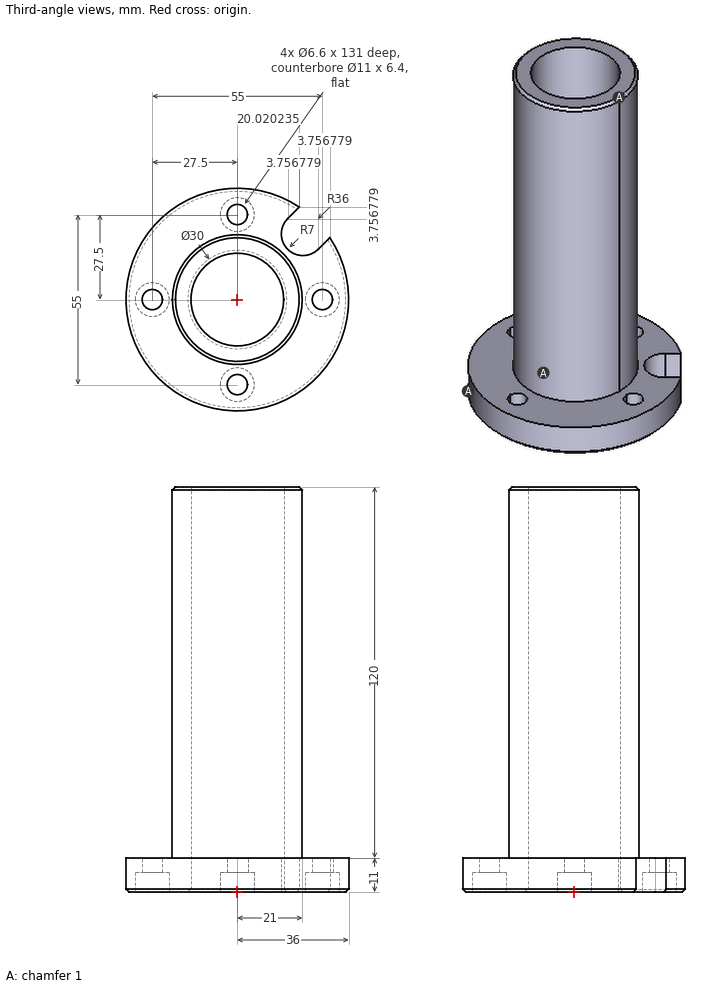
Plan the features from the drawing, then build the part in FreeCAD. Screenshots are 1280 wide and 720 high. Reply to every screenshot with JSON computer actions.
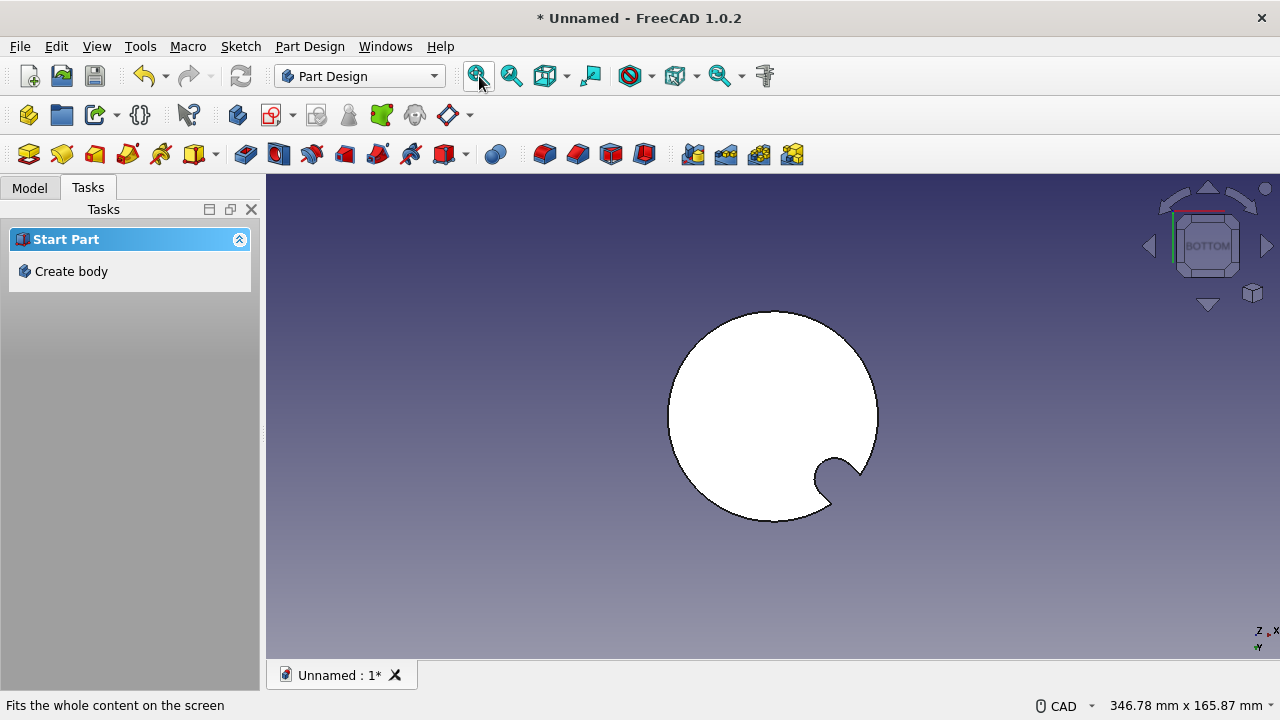
{"action": "left_click", "coordinate": [479, 76]}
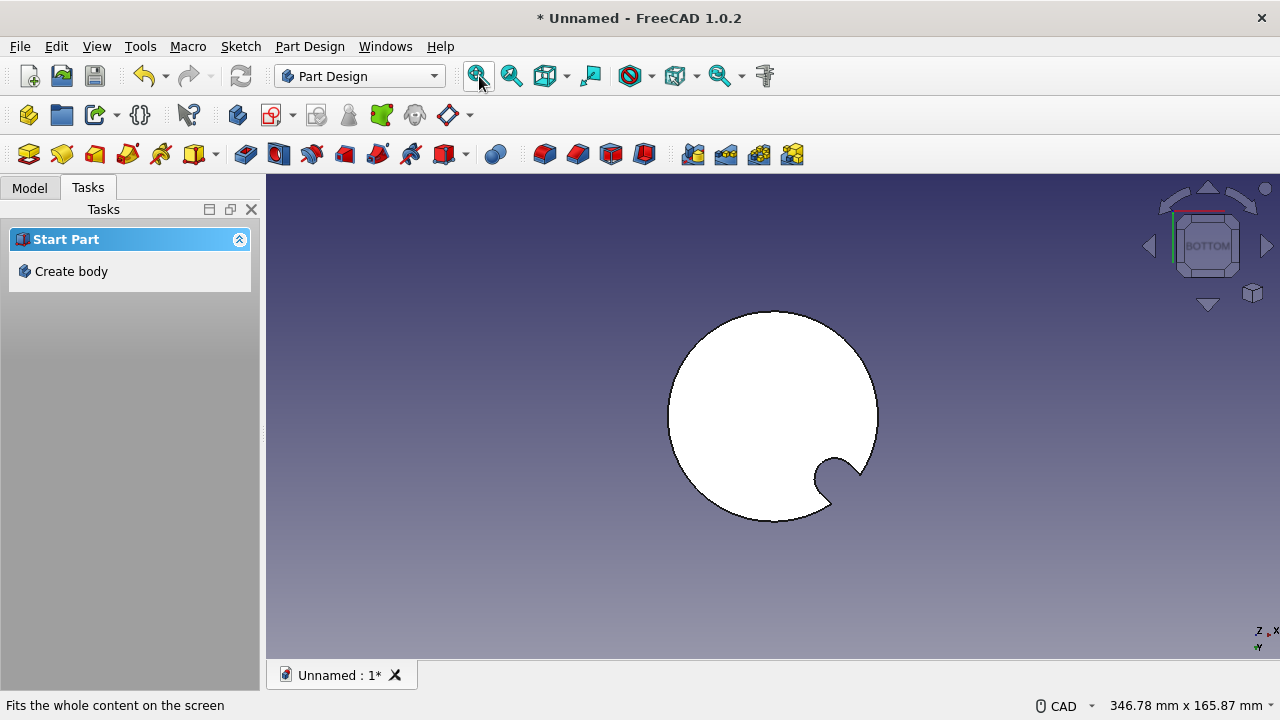
{"action": "left_click", "coordinate": [773, 385]}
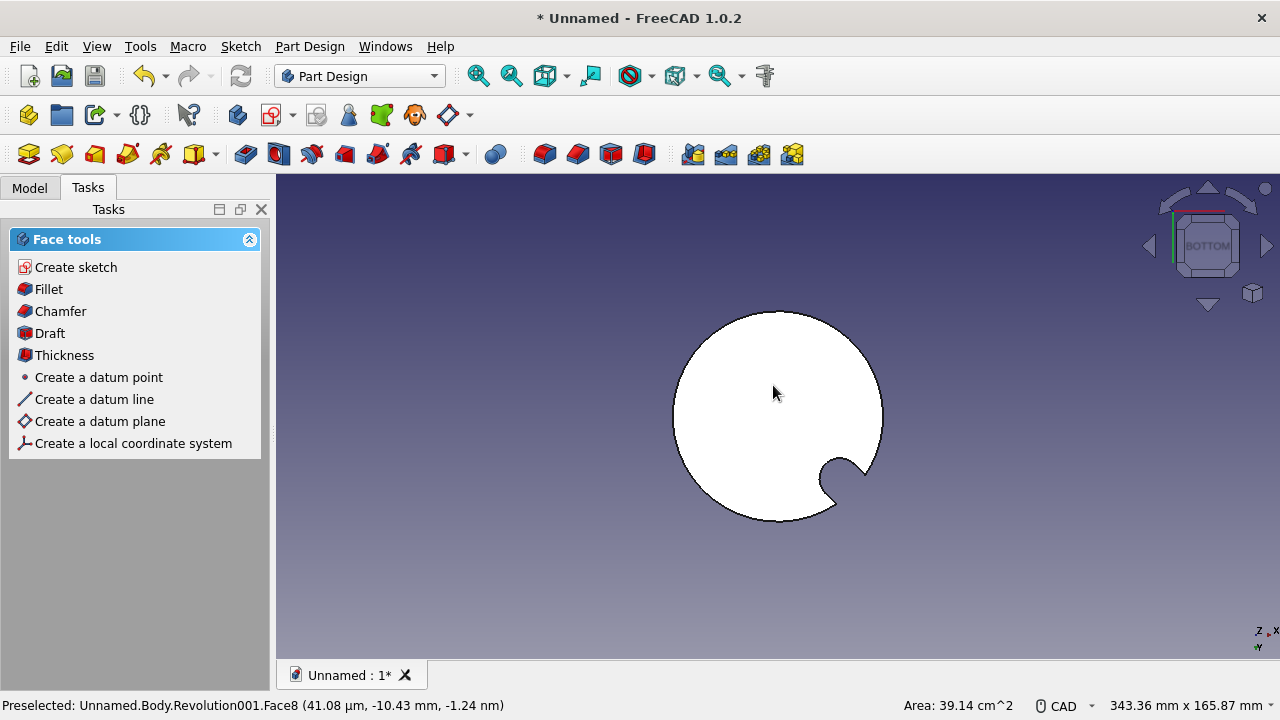
{"action": "left_click", "coordinate": [270, 116]}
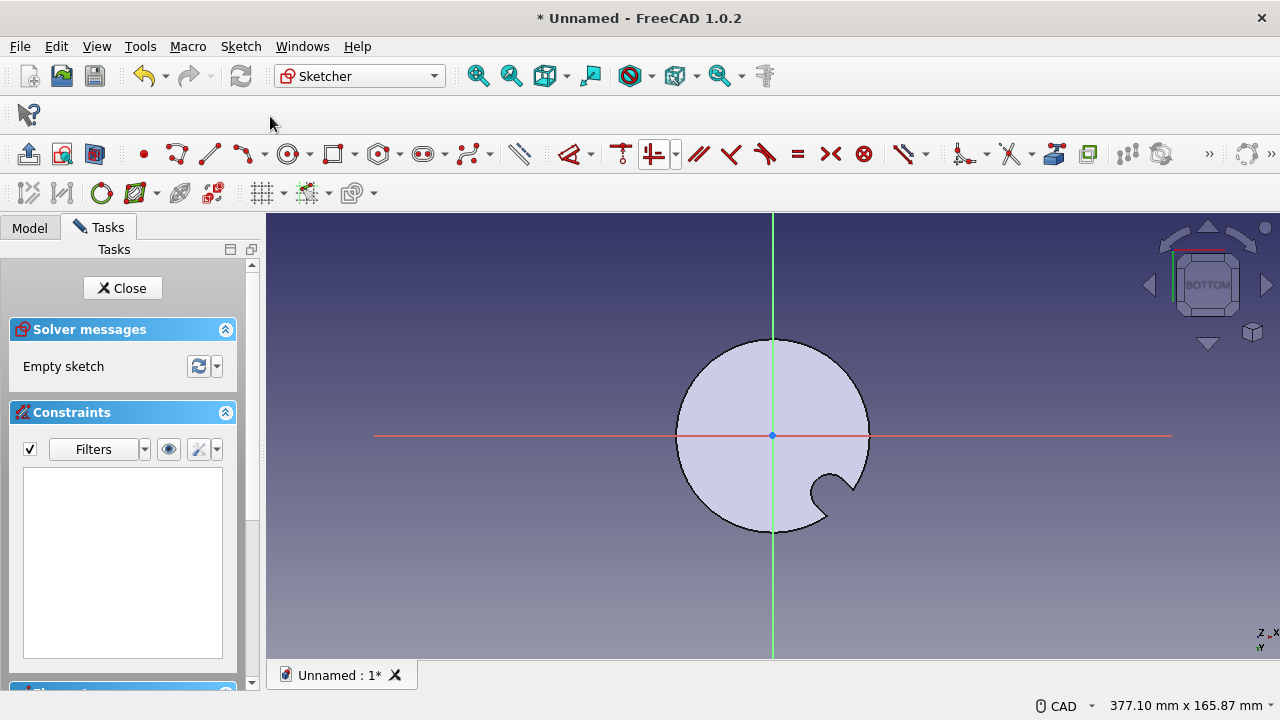
{"action": "scroll", "coordinate": [802, 436], "scroll_direction": "up", "scroll_amount": 6}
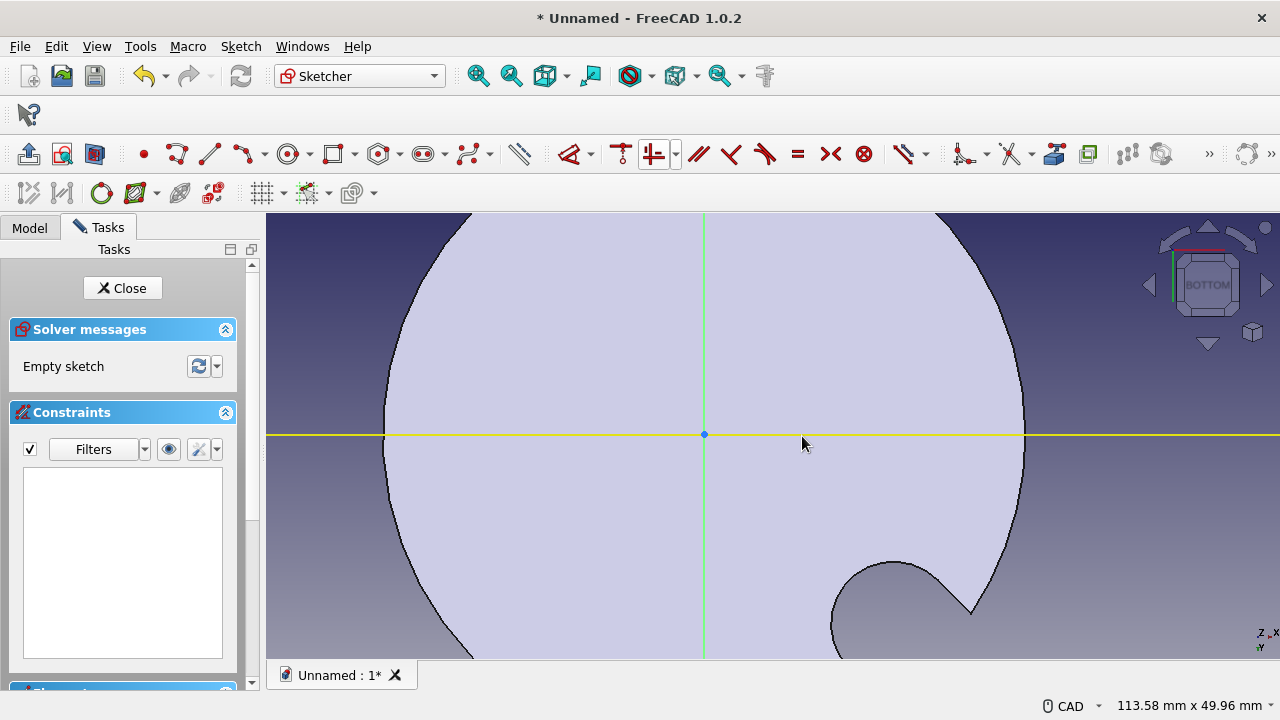
{"action": "left_click", "coordinate": [288, 154]}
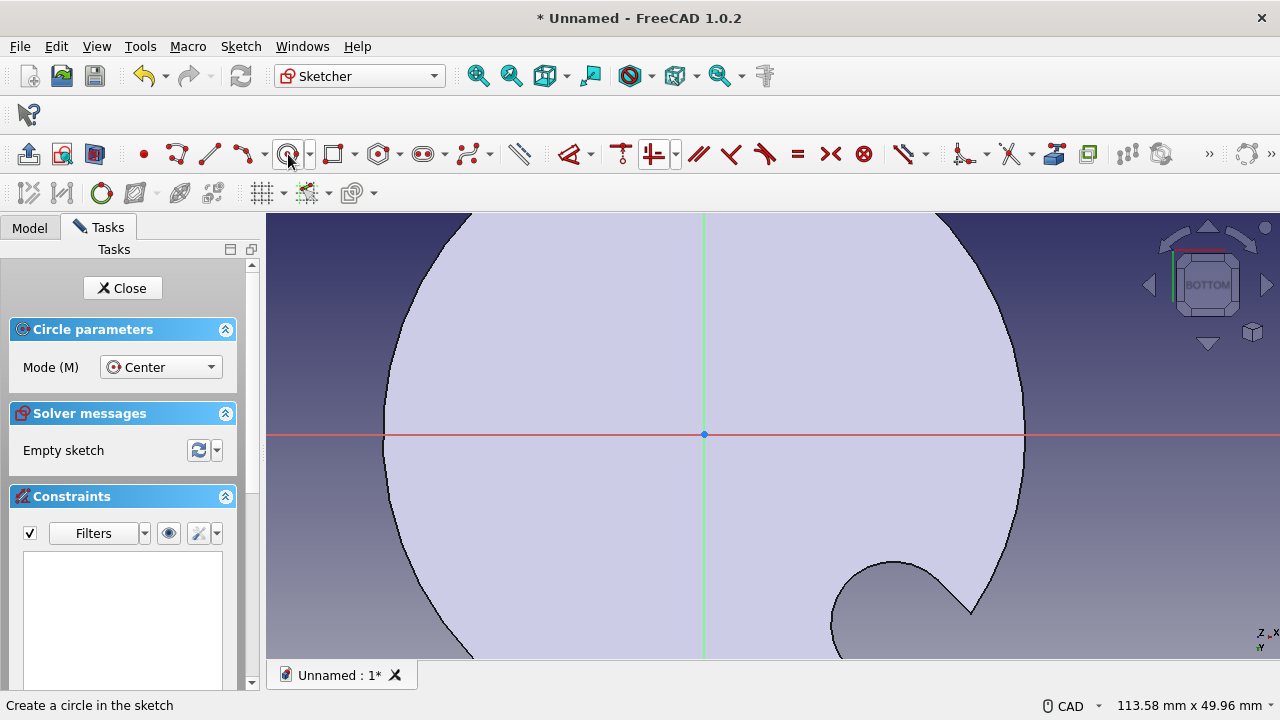
{"action": "left_click", "coordinate": [704, 435]}
{"action": "mouse_move", "coordinate": [799, 340]}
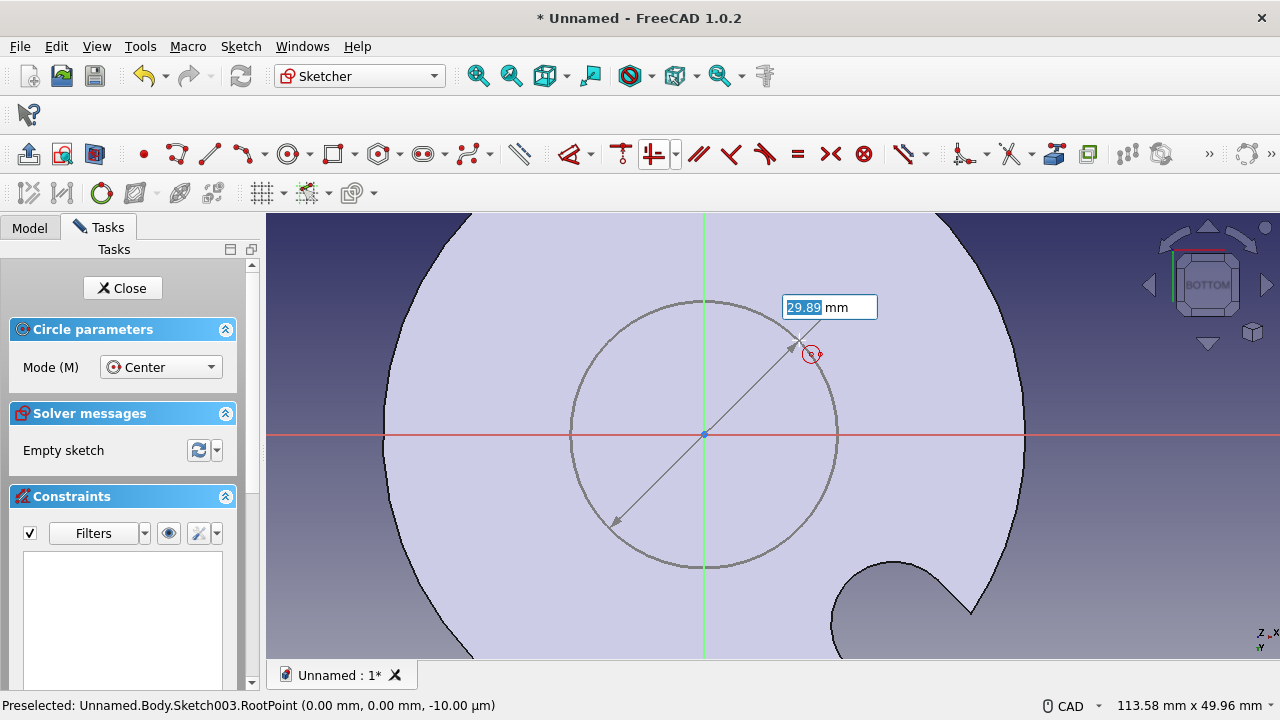
{"action": "type", "text": "30"}
{"action": "key", "text": "Return"}
{"action": "key", "text": "Escape"}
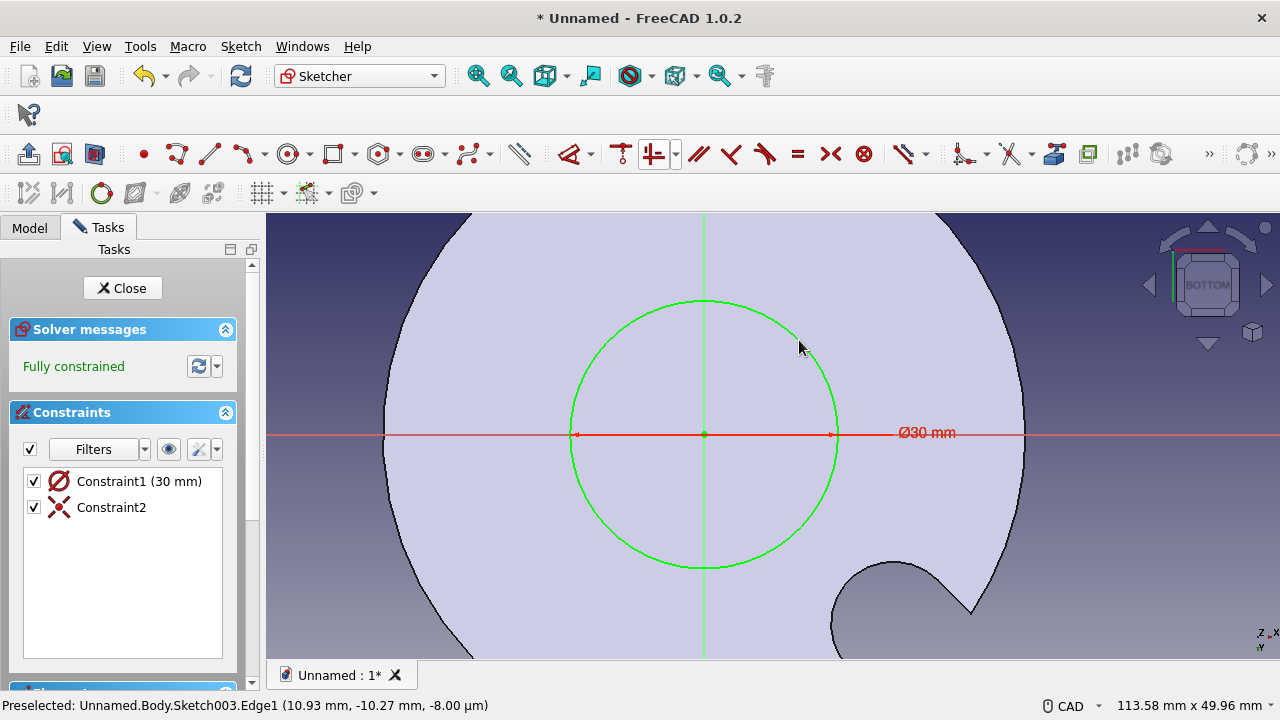
{"action": "left_click", "coordinate": [123, 288]}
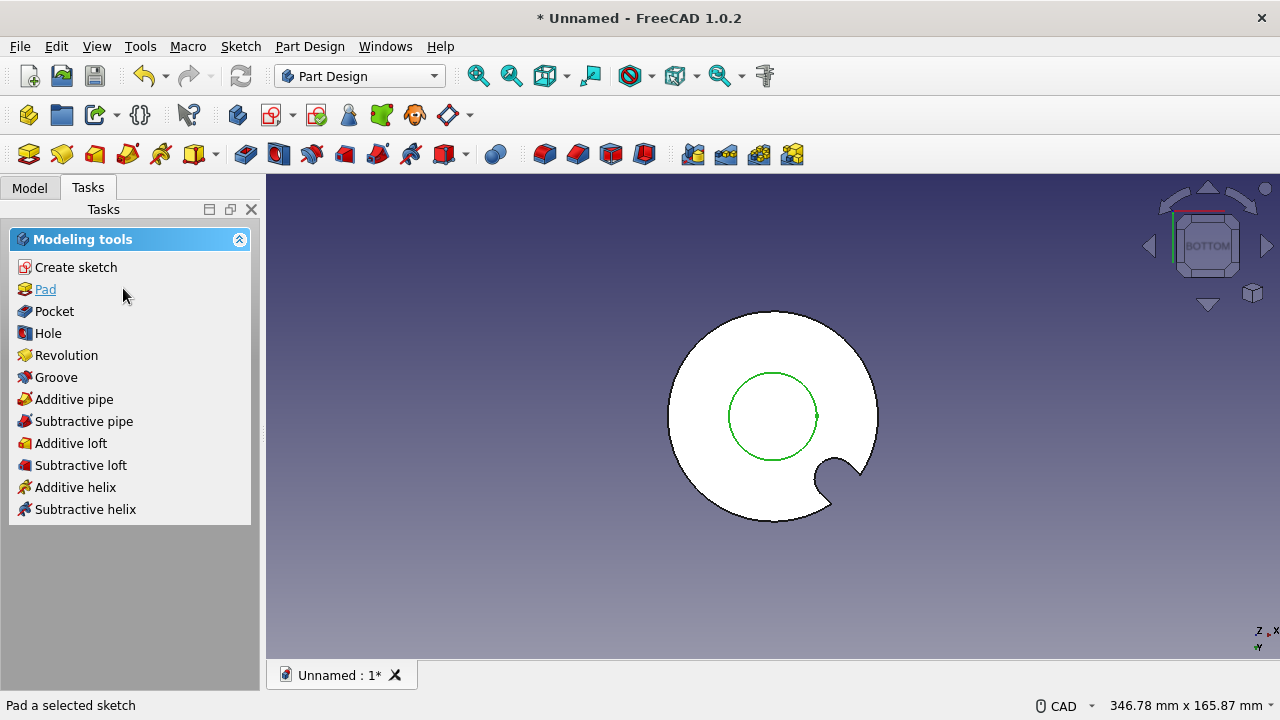
{"action": "left_click", "coordinate": [246, 154]}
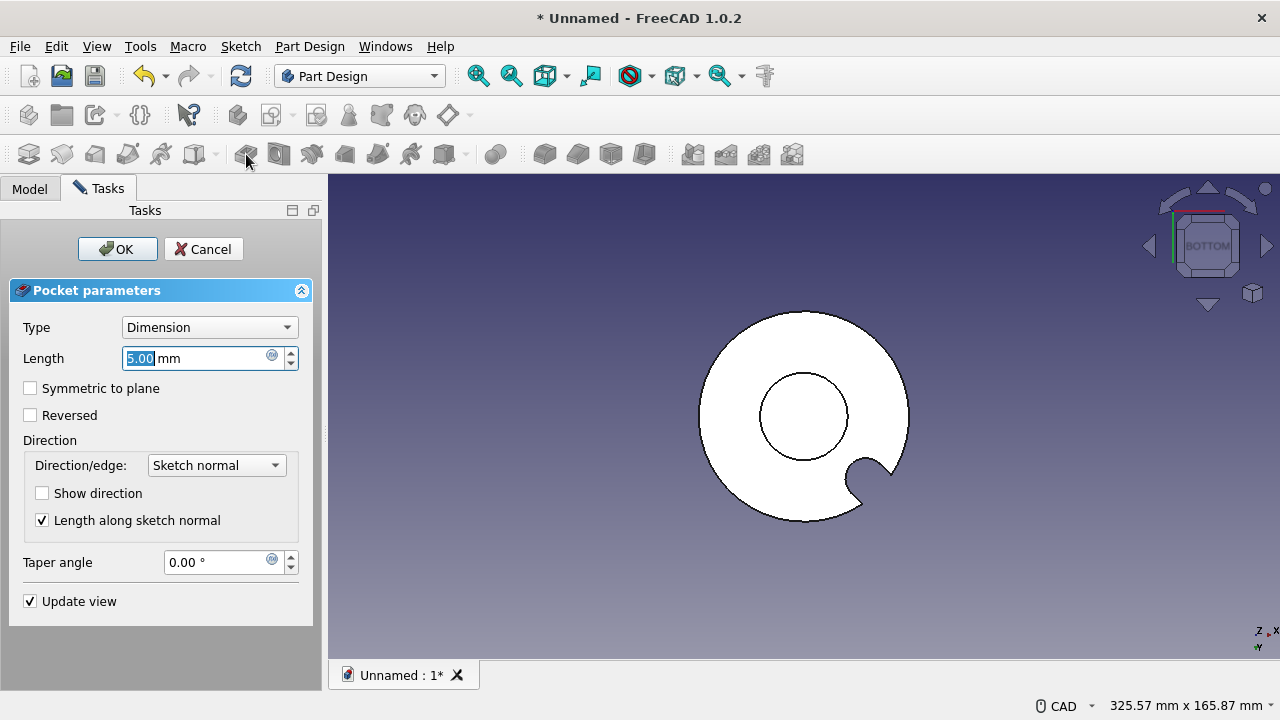
{"action": "left_click", "coordinate": [210, 328]}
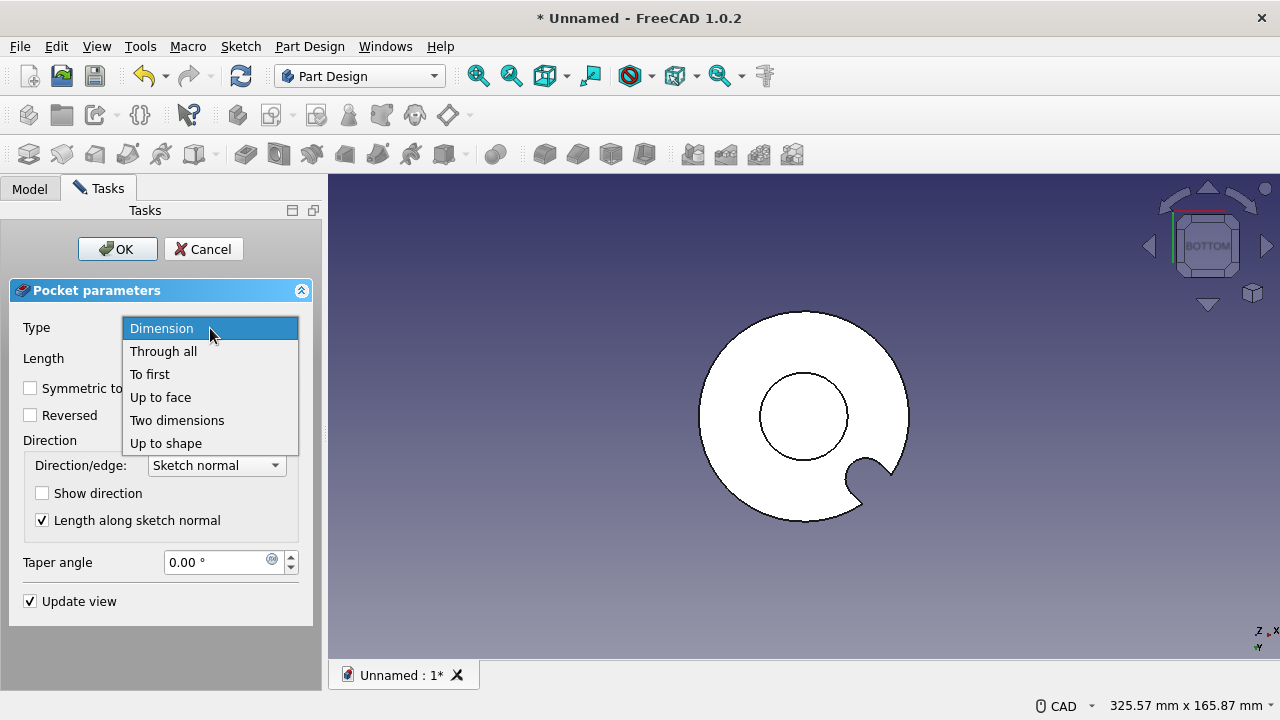
{"action": "left_click", "coordinate": [208, 352]}